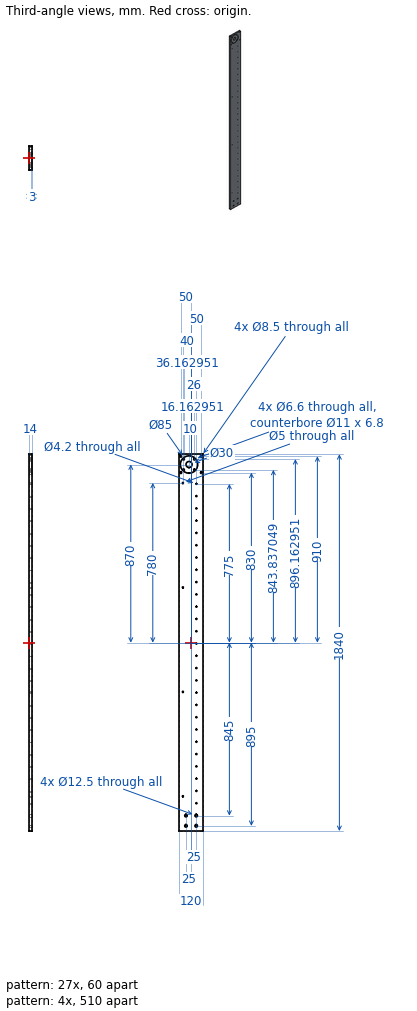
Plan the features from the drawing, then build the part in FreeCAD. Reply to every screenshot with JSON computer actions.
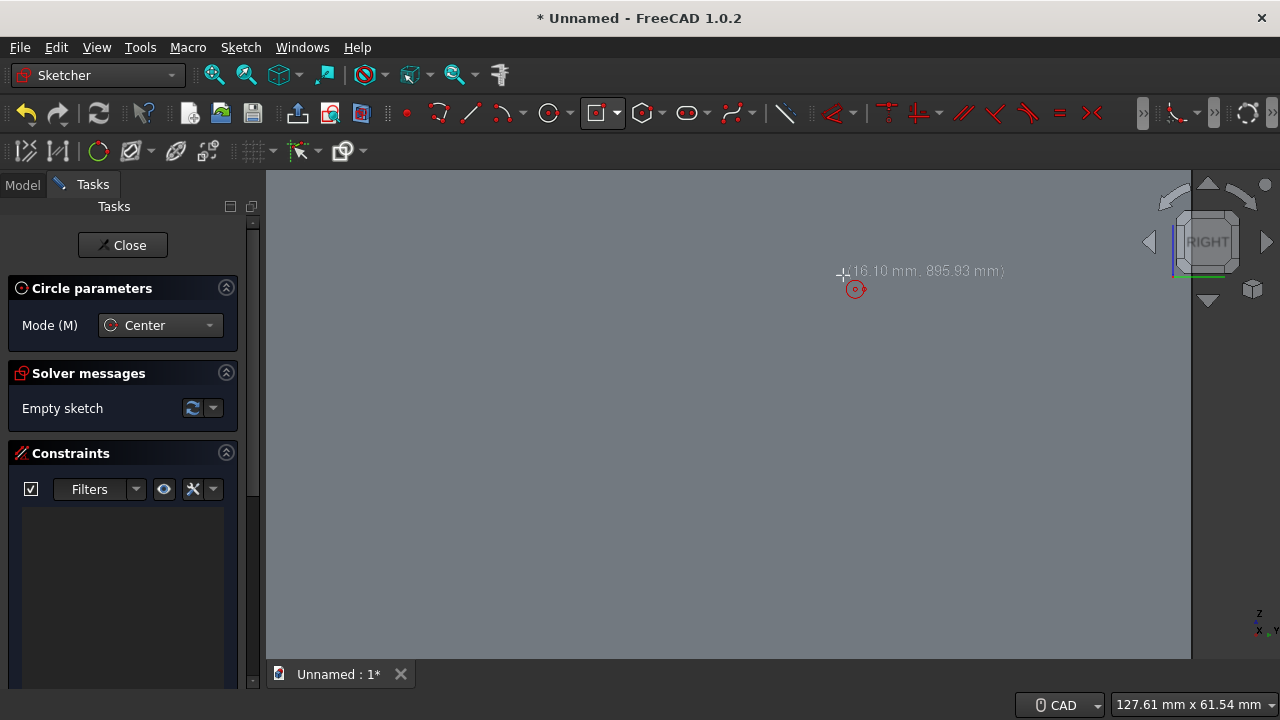
{"action": "left_click", "coordinate": [843, 275]}
{"action": "mouse_move", "coordinate": [862, 256]}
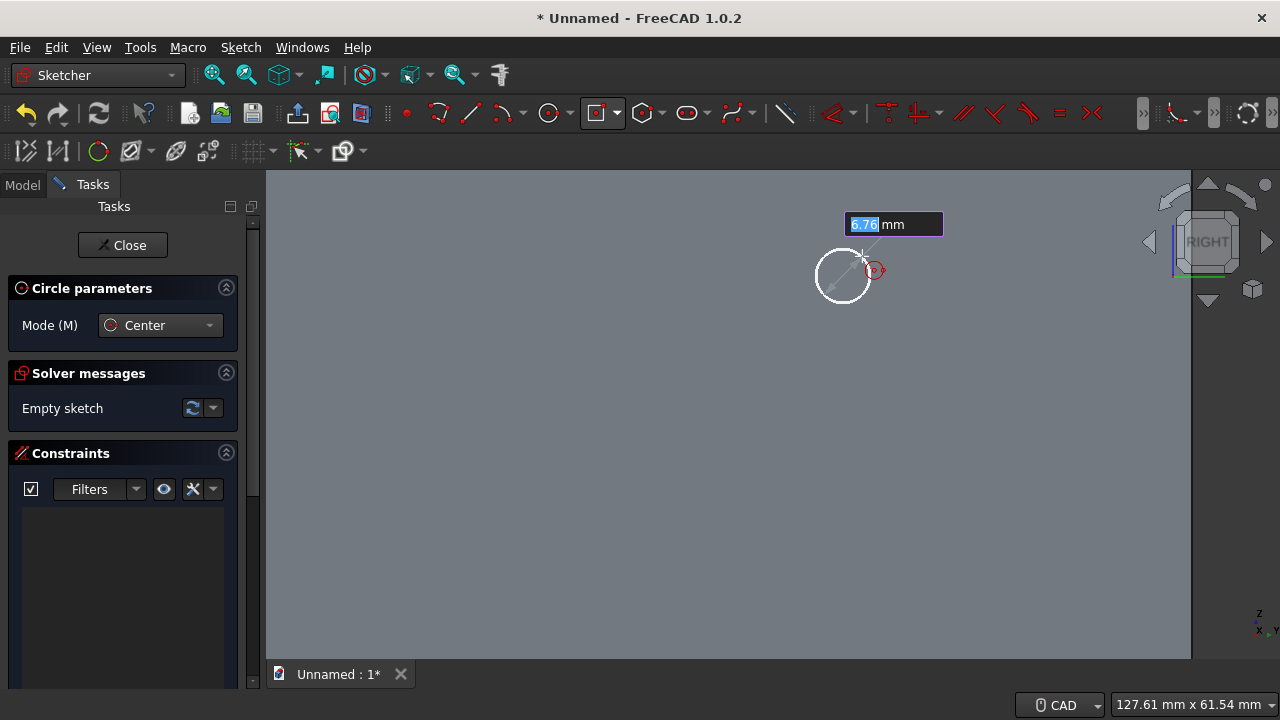
{"action": "type", "text": "6.6"}
{"action": "key", "text": "Return"}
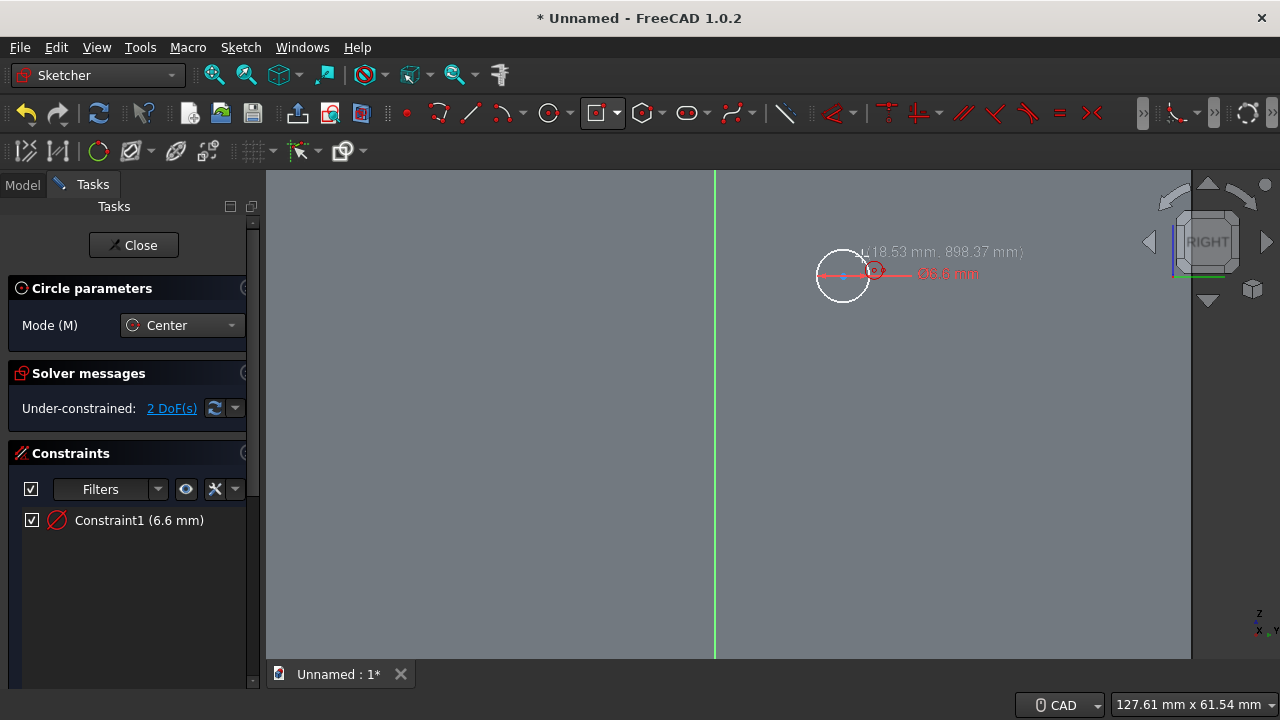
{"action": "scroll", "coordinate": [845, 276], "scroll_direction": "down", "scroll_amount": 2}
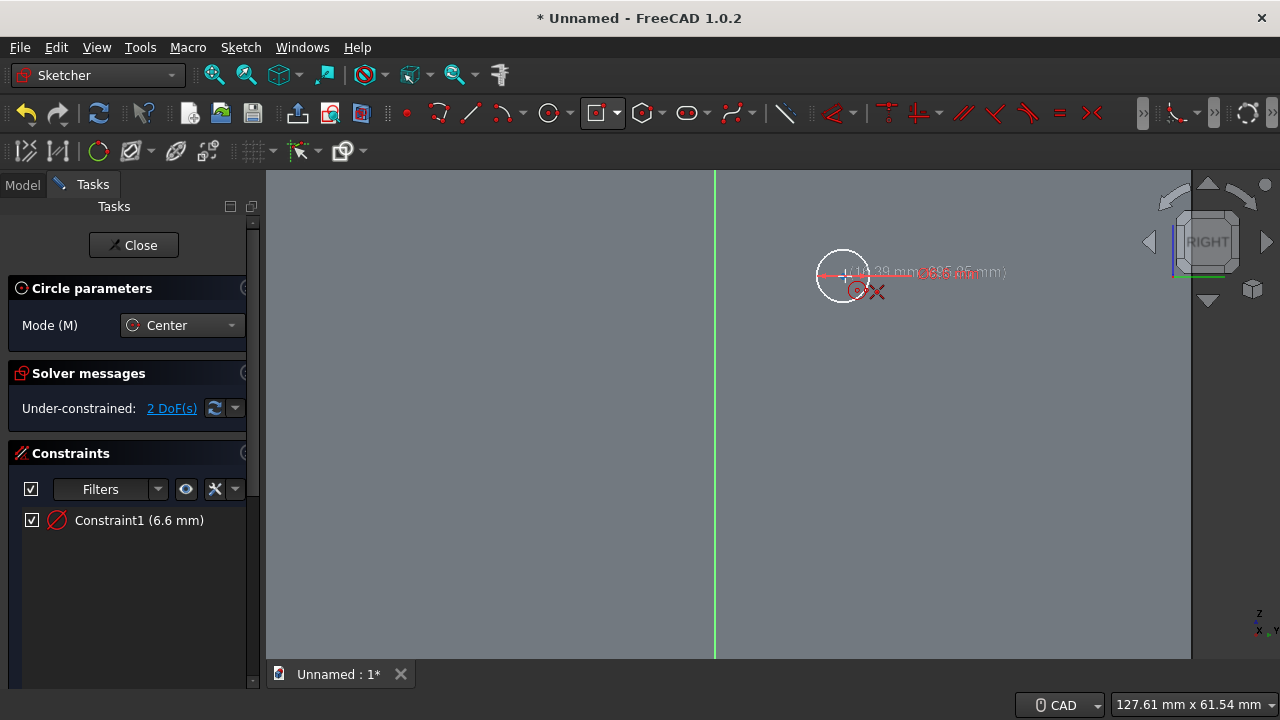
{"action": "scroll", "coordinate": [844, 554], "scroll_direction": "up", "scroll_amount": 2}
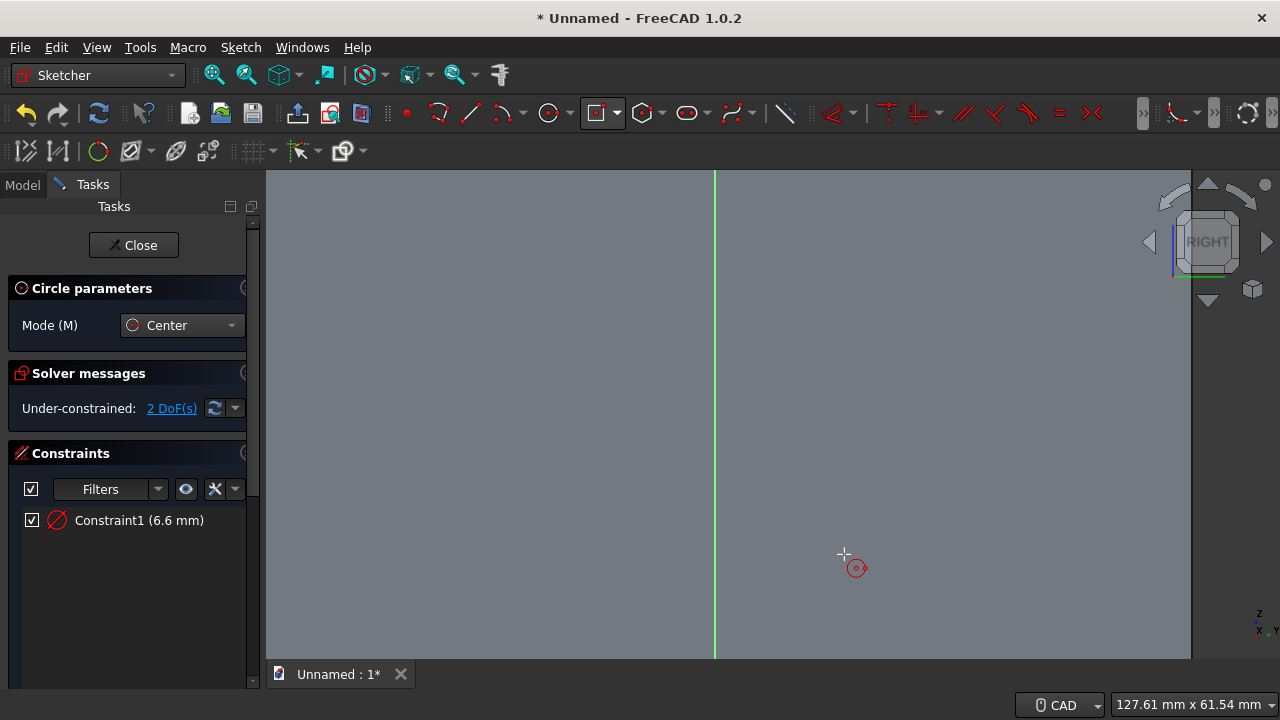
{"action": "left_click", "coordinate": [844, 553]}
{"action": "mouse_move", "coordinate": [862, 535]}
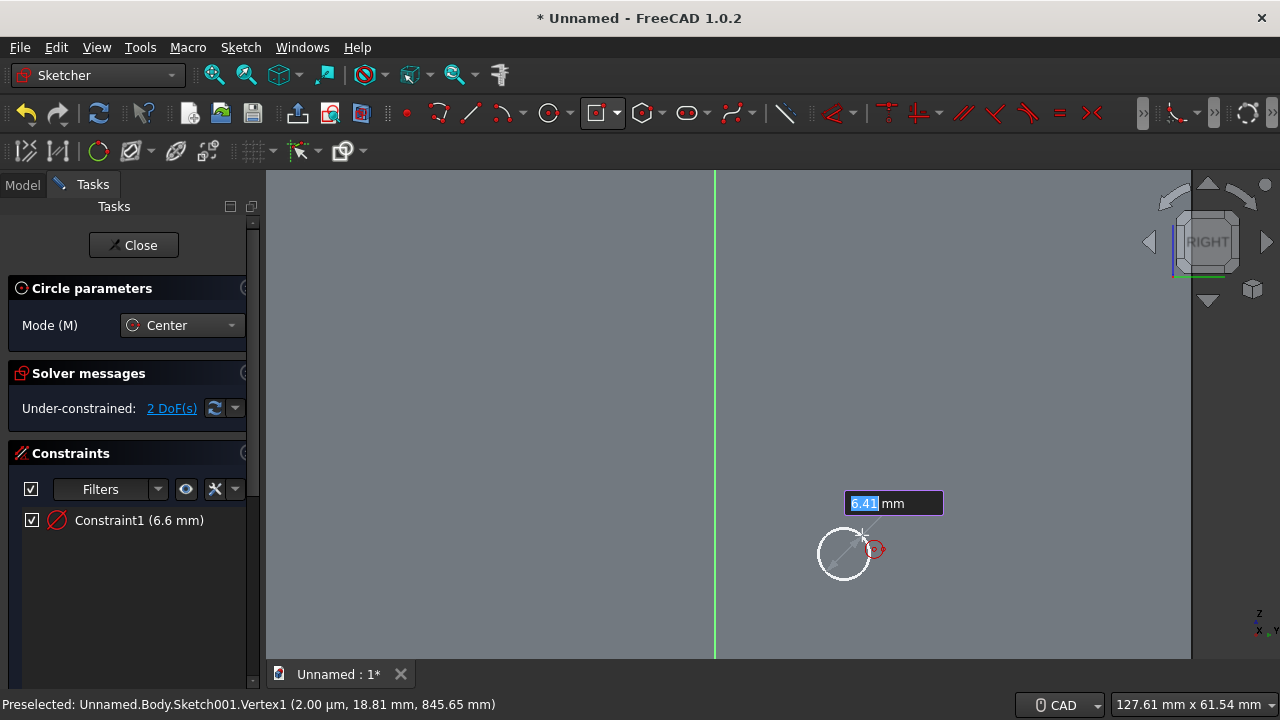
{"action": "type", "text": "6.6"}
{"action": "key", "text": "Return"}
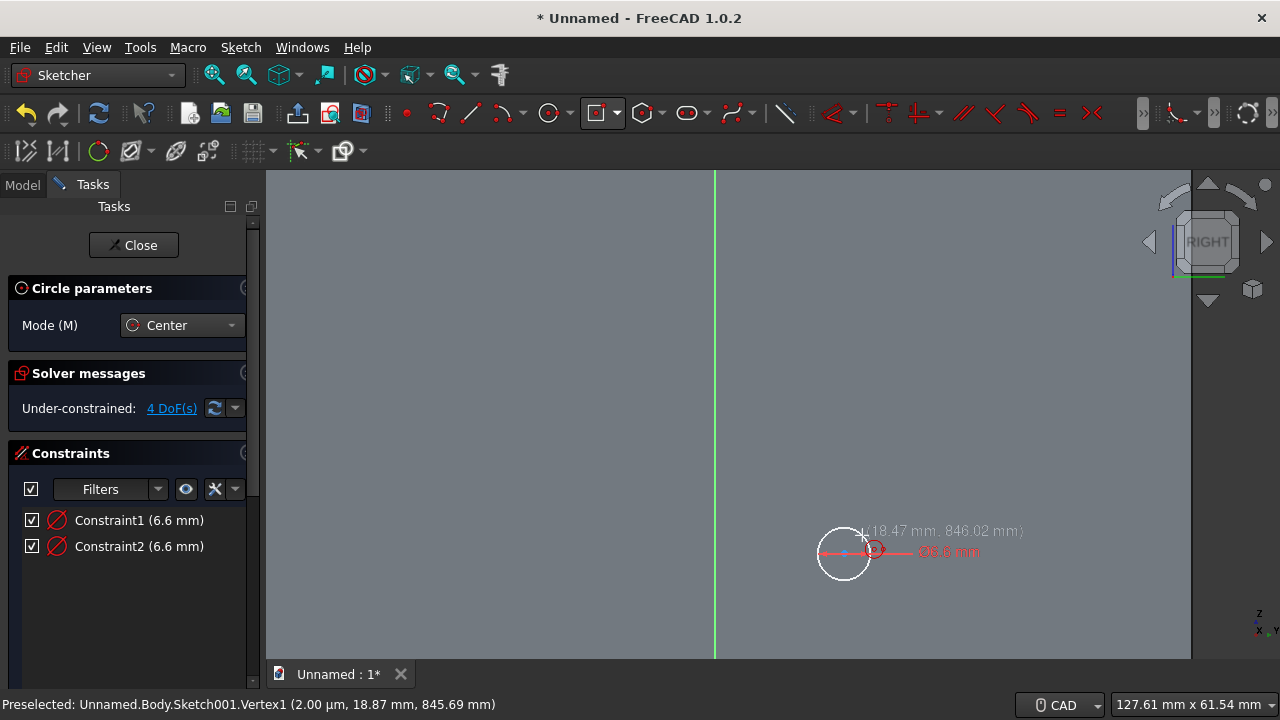
{"action": "scroll", "coordinate": [844, 555], "scroll_direction": "down", "scroll_amount": 2}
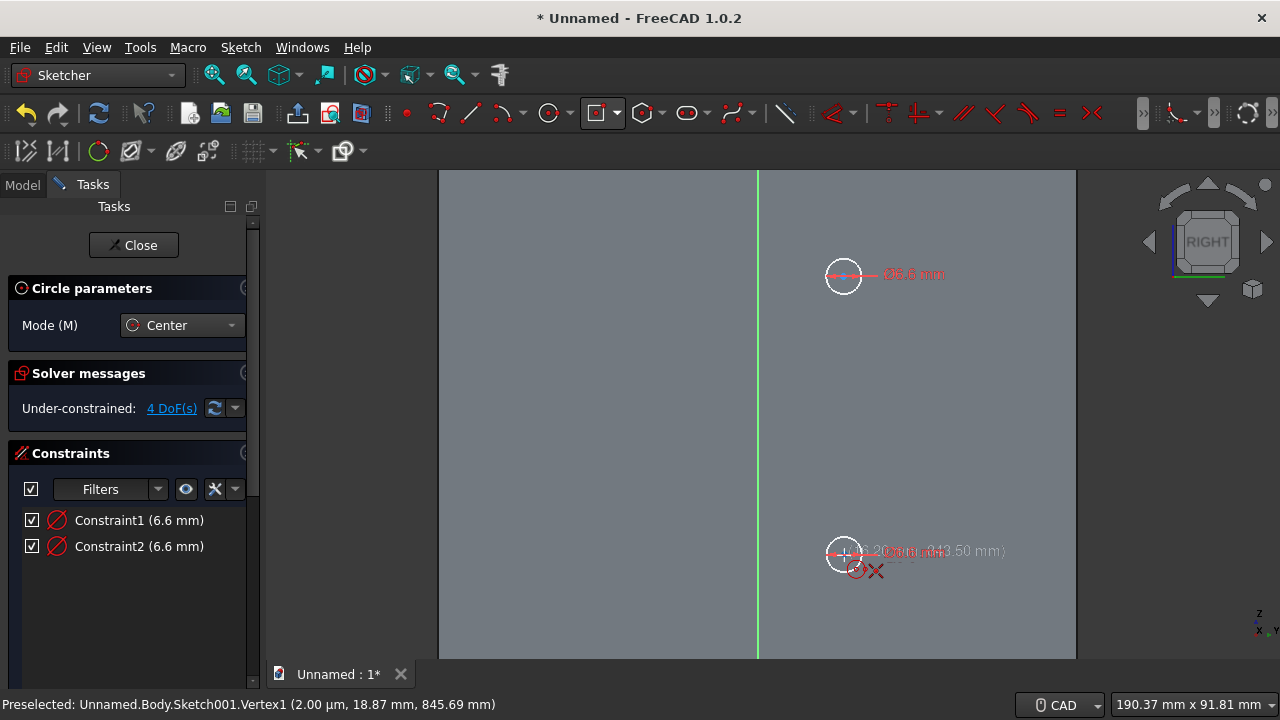
{"action": "scroll", "coordinate": [565, 275], "scroll_direction": "up", "scroll_amount": 2}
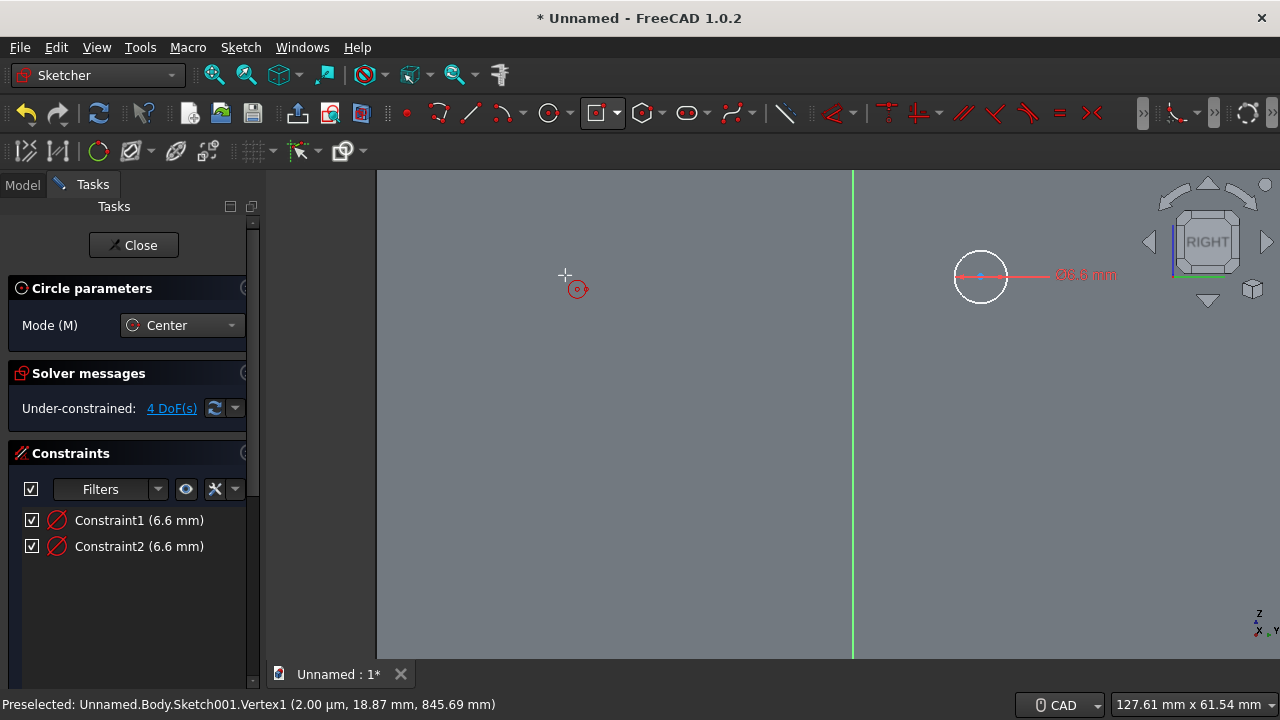
{"action": "left_click", "coordinate": [565, 276]}
{"action": "mouse_move", "coordinate": [584, 257]}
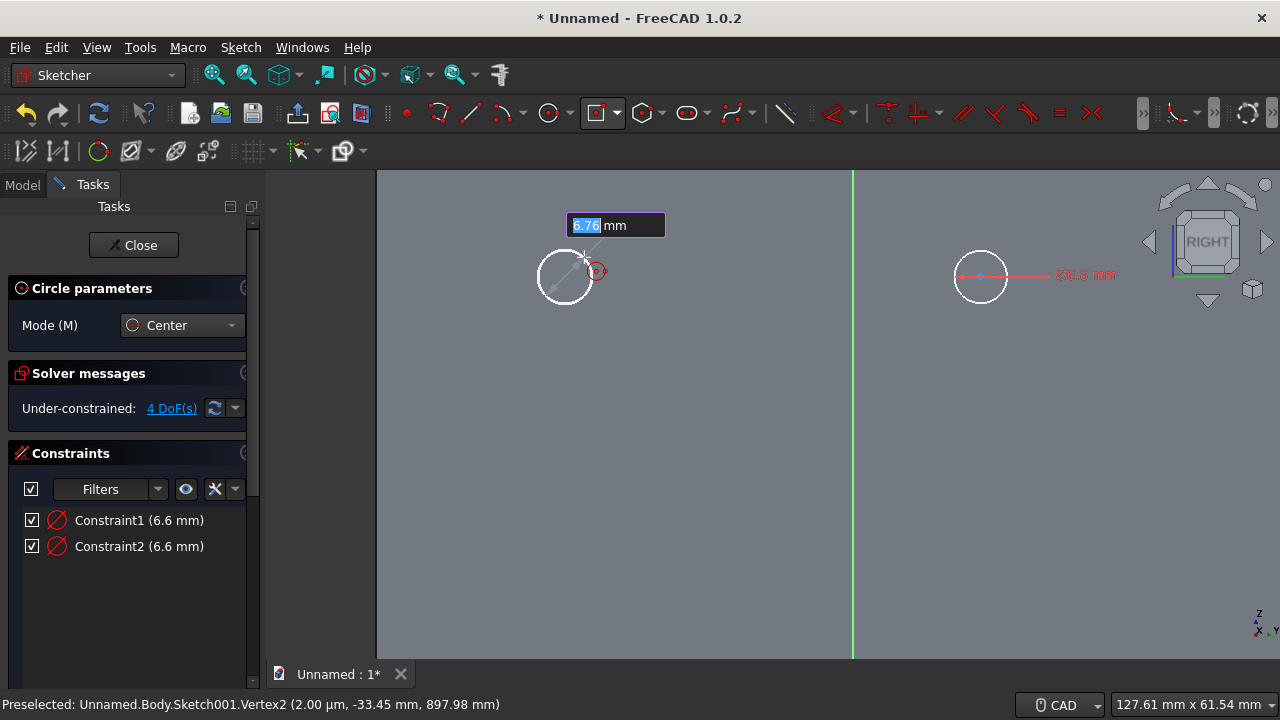
{"action": "type", "text": "6.6"}
{"action": "key", "text": "Return"}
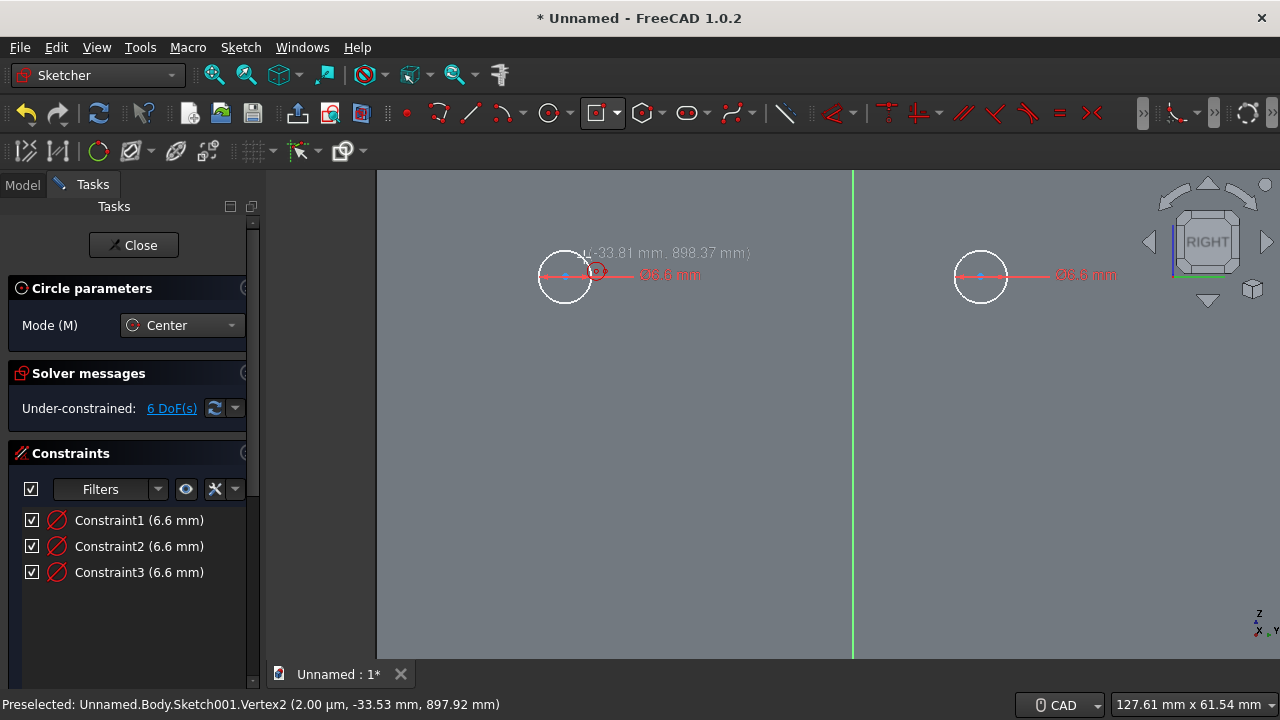
{"action": "scroll", "coordinate": [565, 274], "scroll_direction": "down", "scroll_amount": 2}